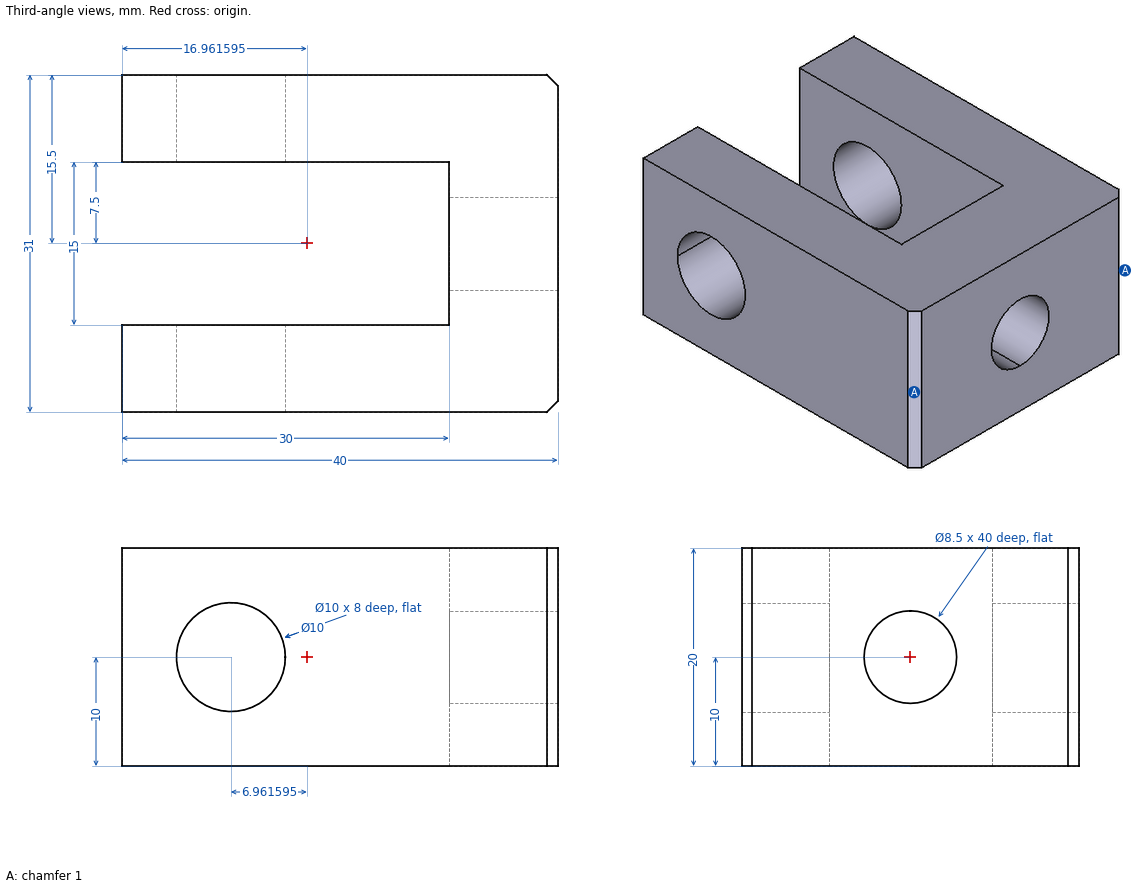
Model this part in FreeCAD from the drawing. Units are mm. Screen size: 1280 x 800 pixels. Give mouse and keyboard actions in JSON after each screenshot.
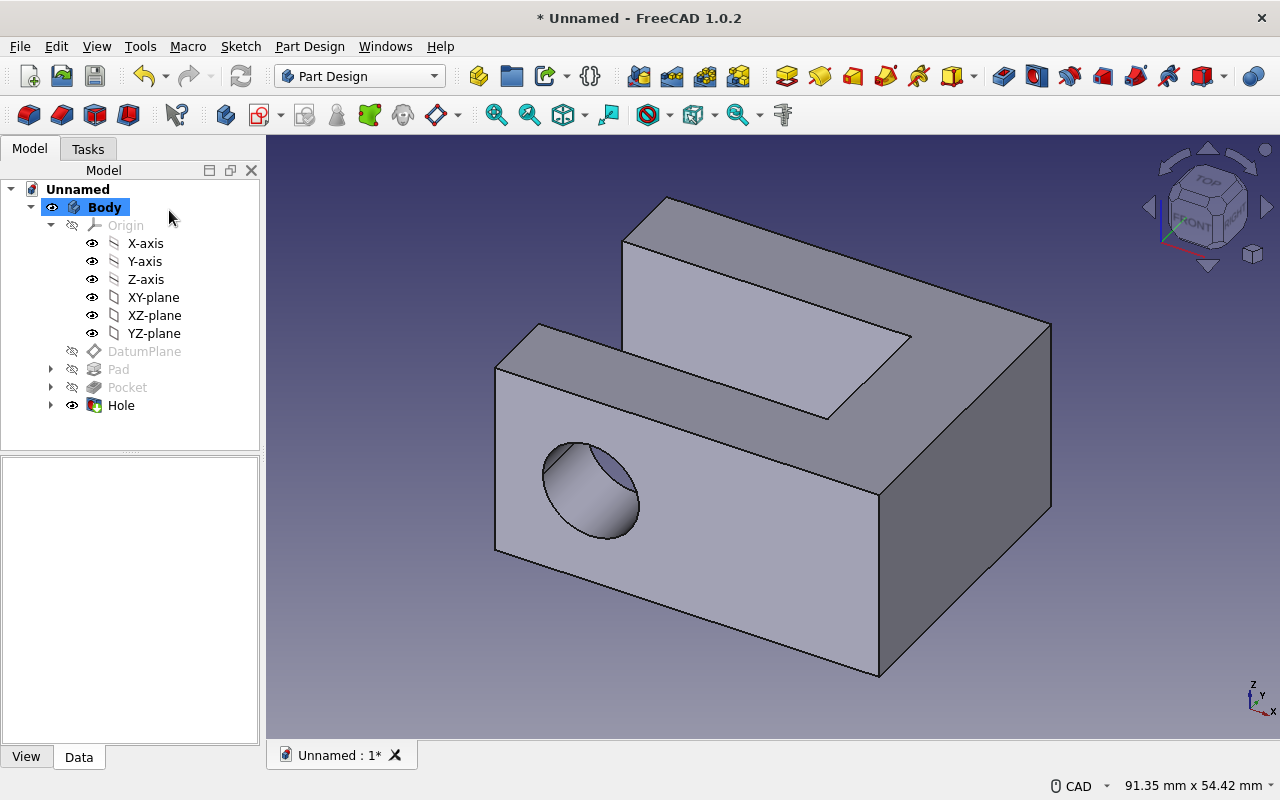
{"action": "left_click", "coordinate": [990, 475]}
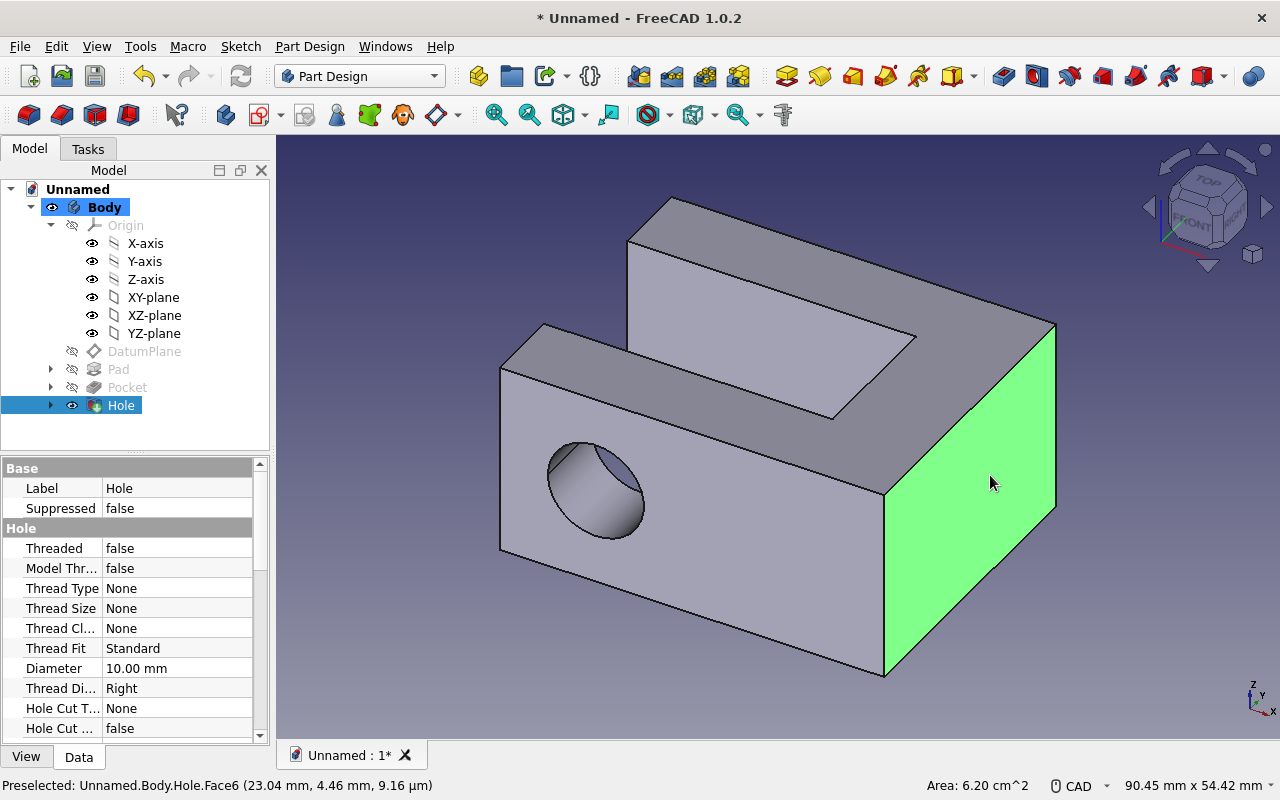
{"action": "left_click", "coordinate": [258, 116]}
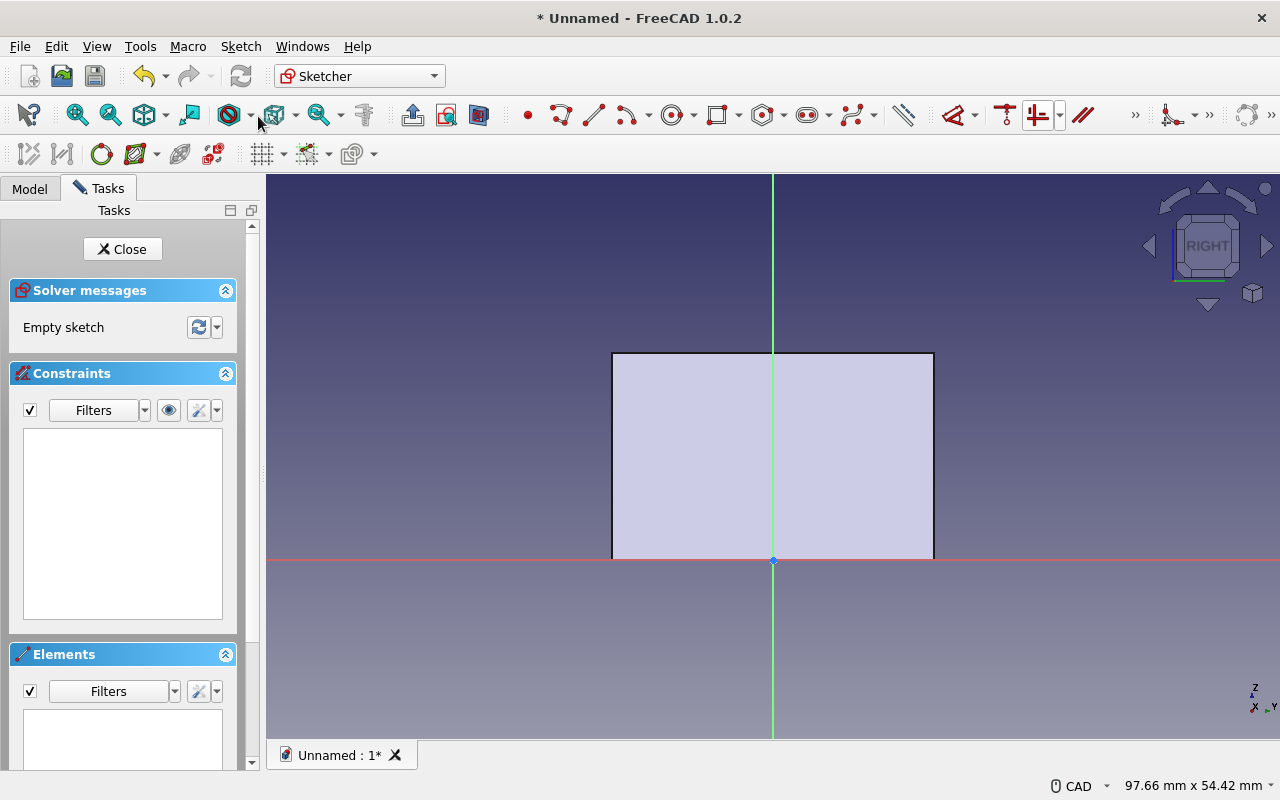
{"action": "scroll", "coordinate": [829, 511], "scroll_direction": "up", "scroll_amount": 4}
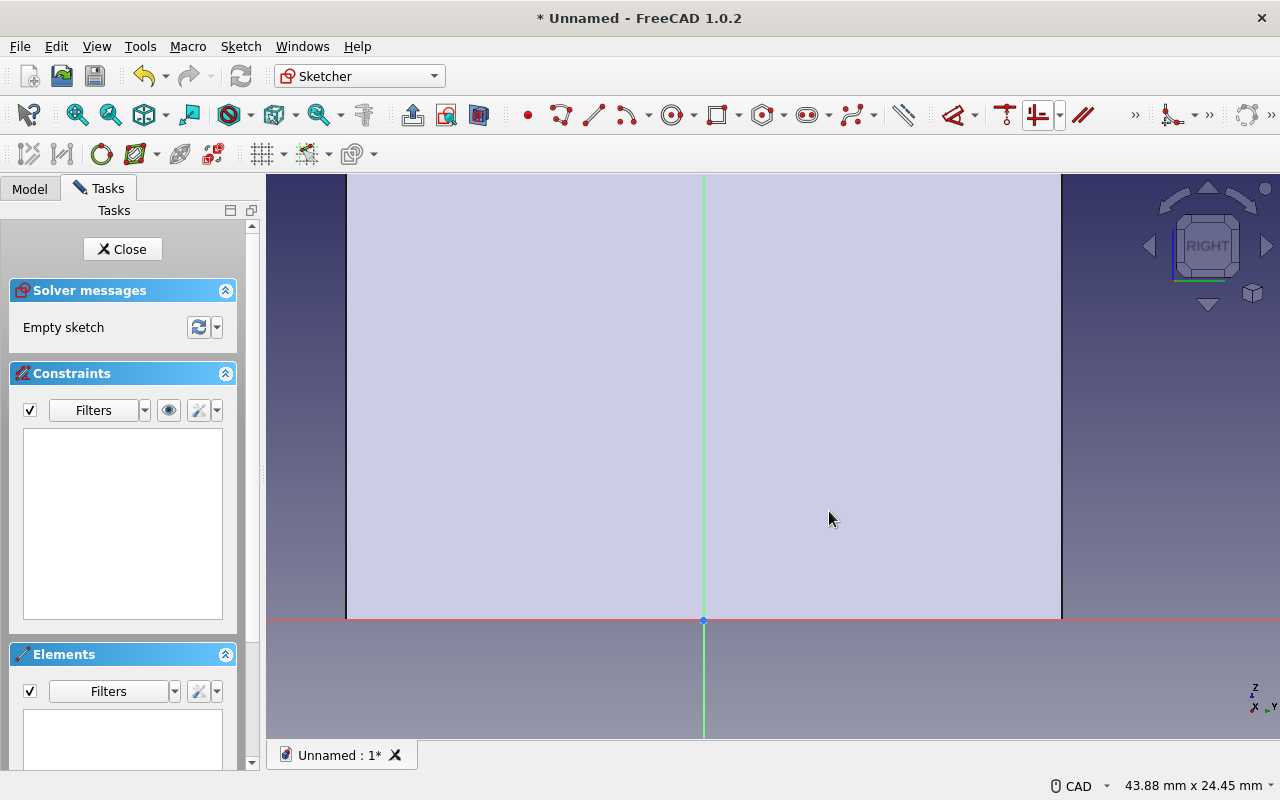
{"action": "left_click", "coordinate": [672, 116]}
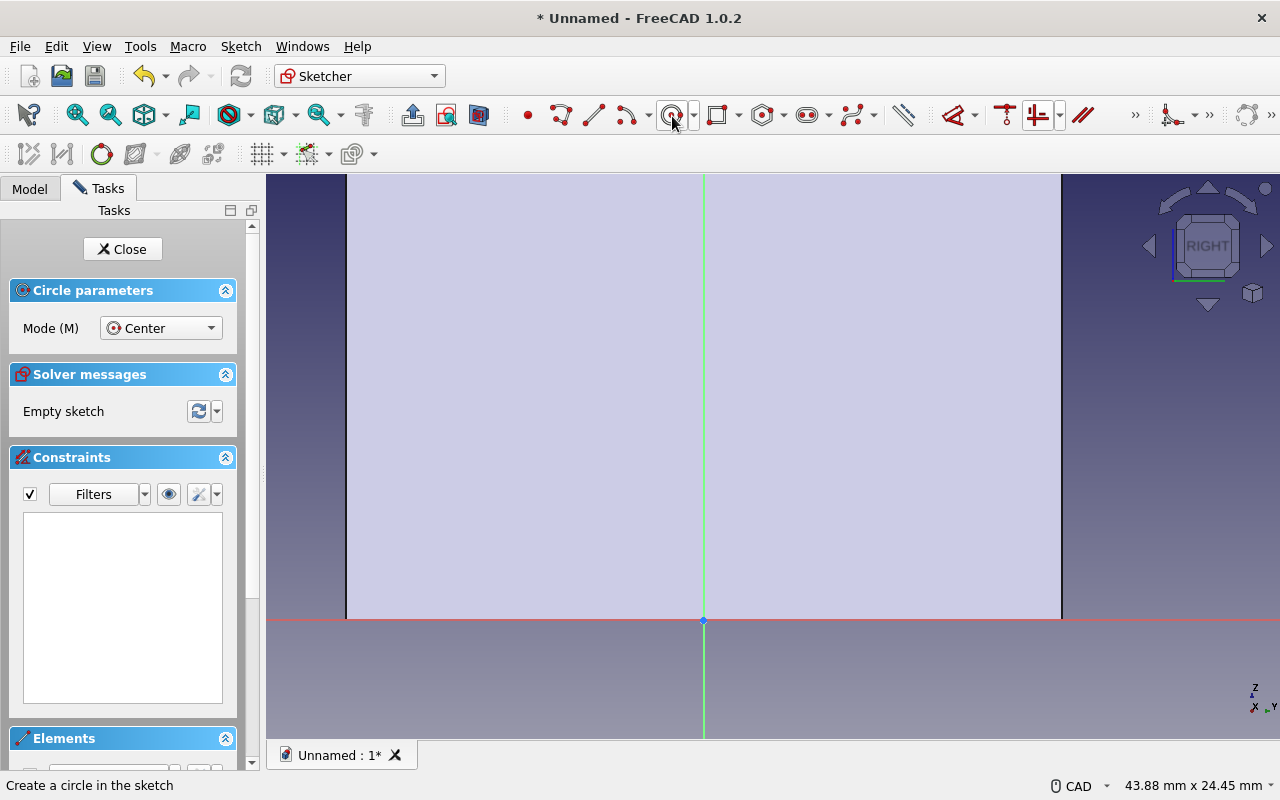
{"action": "left_click", "coordinate": [704, 389]}
{"action": "left_click", "coordinate": [773, 320]}
{"action": "key", "text": "Escape"}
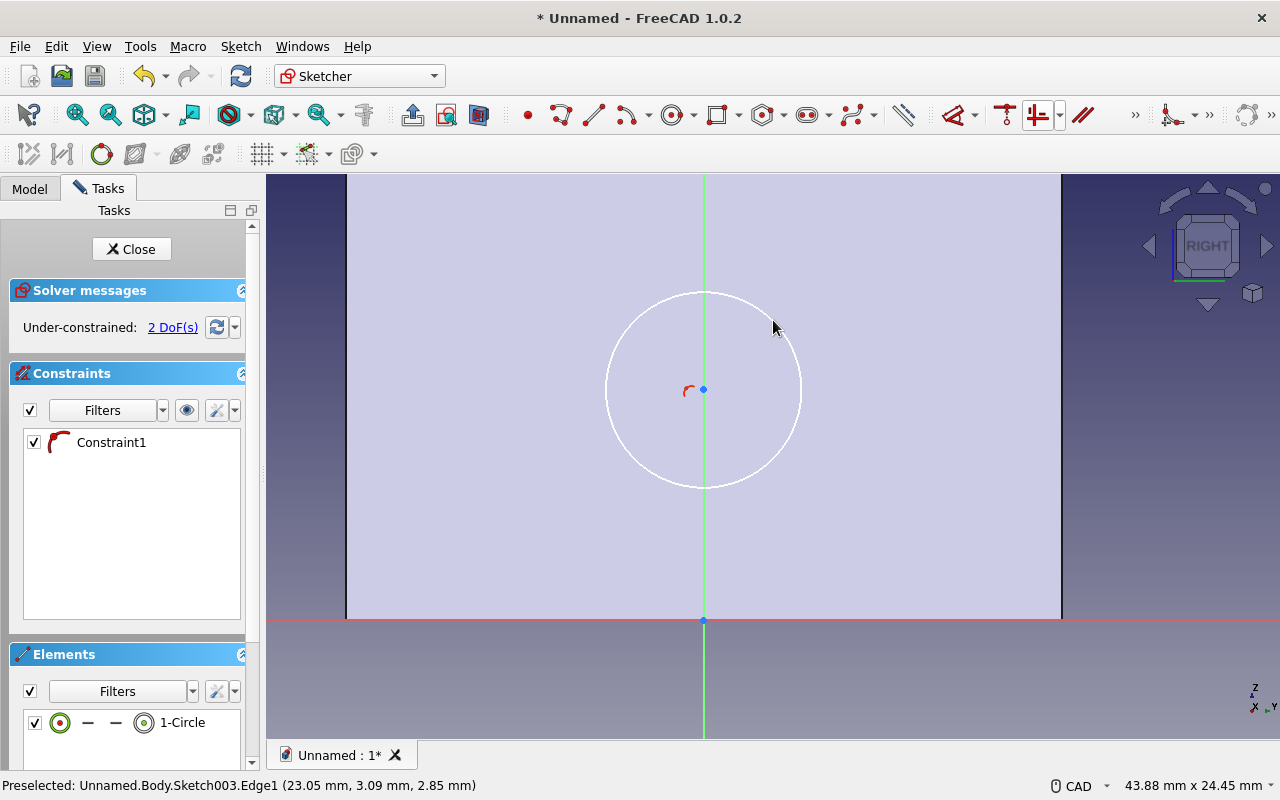
{"action": "key", "text": "d"}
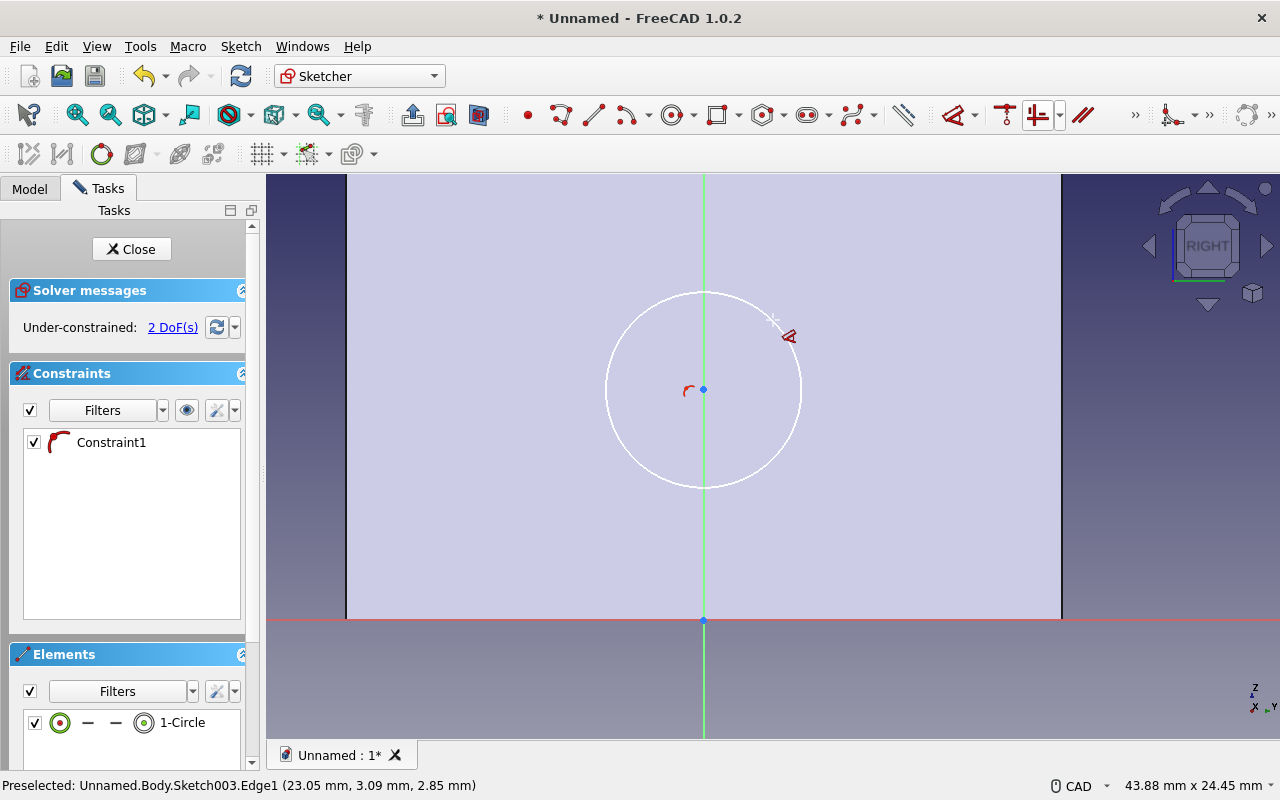
{"action": "left_click", "coordinate": [773, 321]}
{"action": "left_click", "coordinate": [796, 298]}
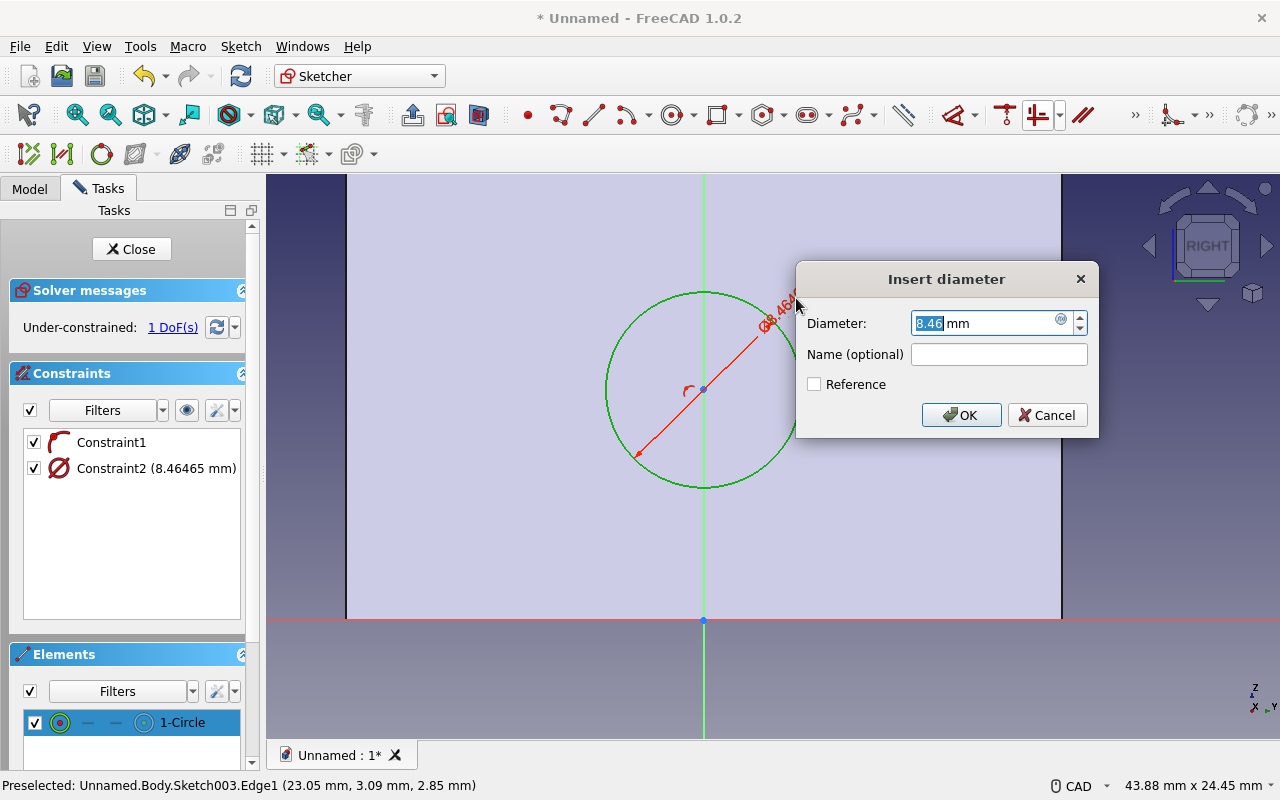
{"action": "type", "text": "8.5"}
{"action": "key", "text": "Return"}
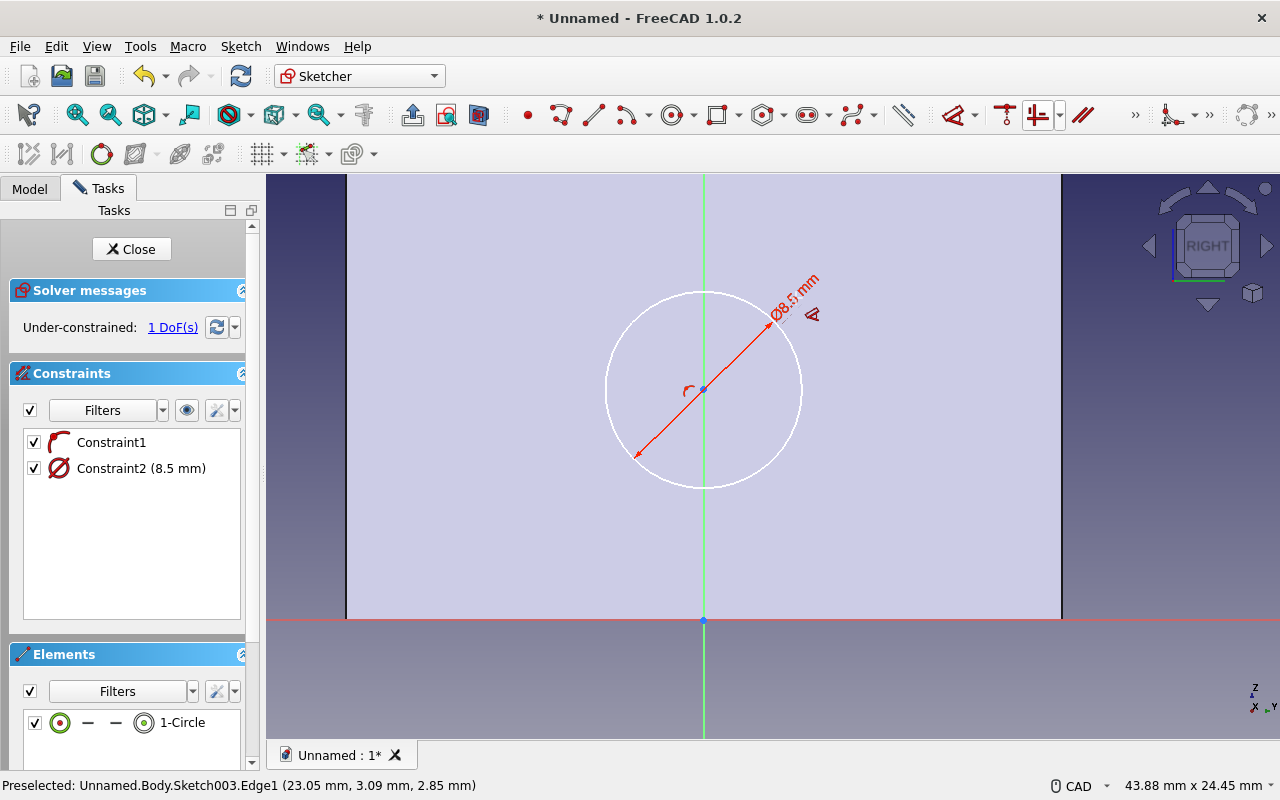
{"action": "left_click", "coordinate": [704, 390]}
{"action": "left_click", "coordinate": [738, 505]}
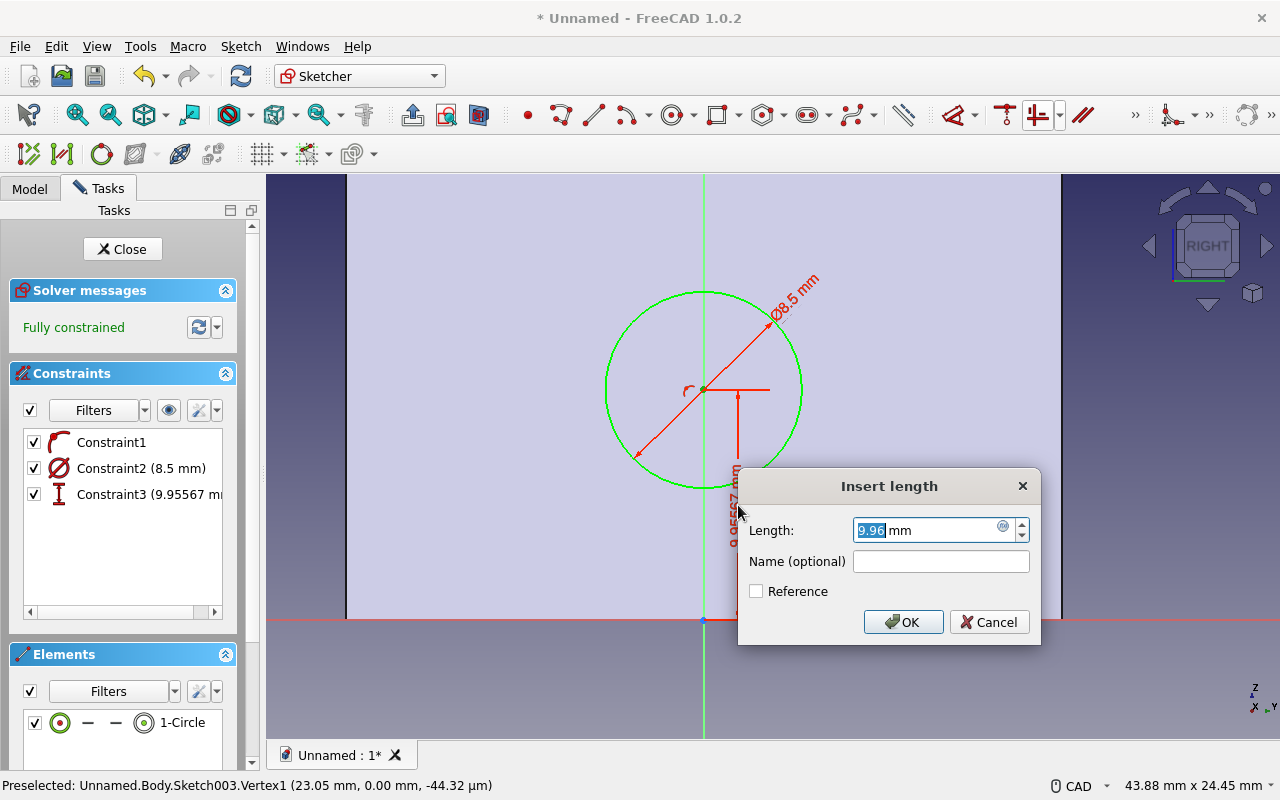
{"action": "type", "text": "10"}
{"action": "key", "text": "Return"}
{"action": "key", "text": "Escape"}